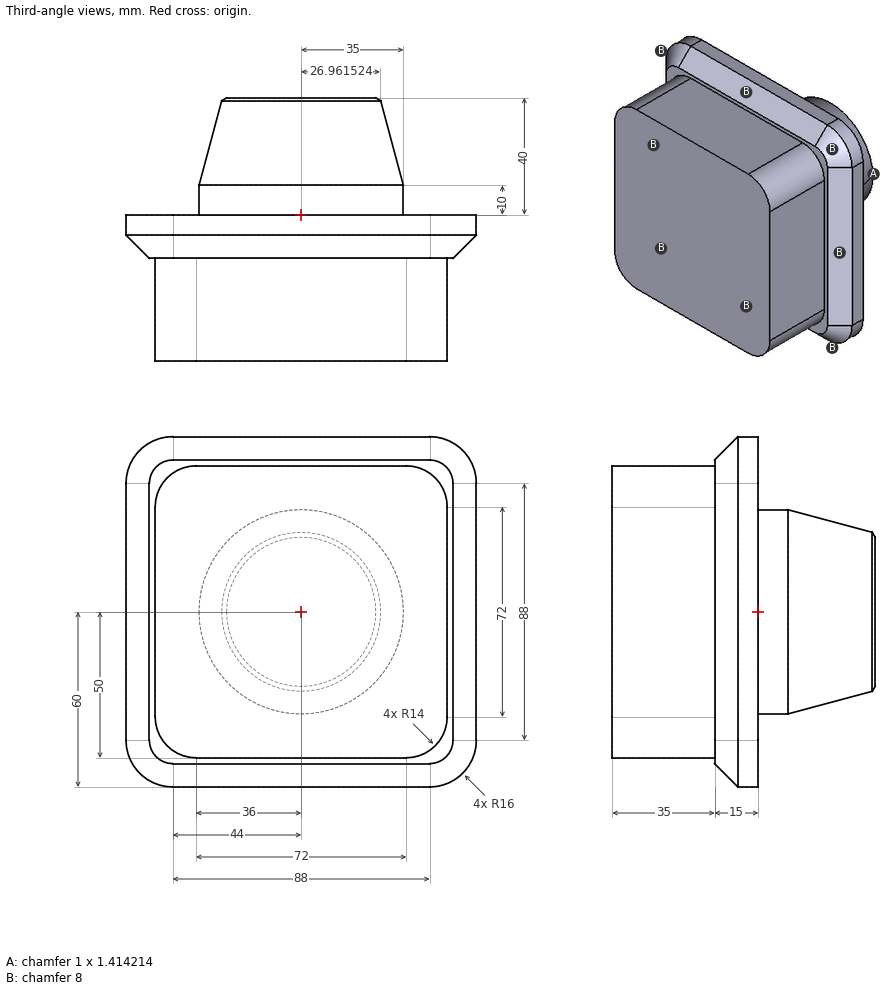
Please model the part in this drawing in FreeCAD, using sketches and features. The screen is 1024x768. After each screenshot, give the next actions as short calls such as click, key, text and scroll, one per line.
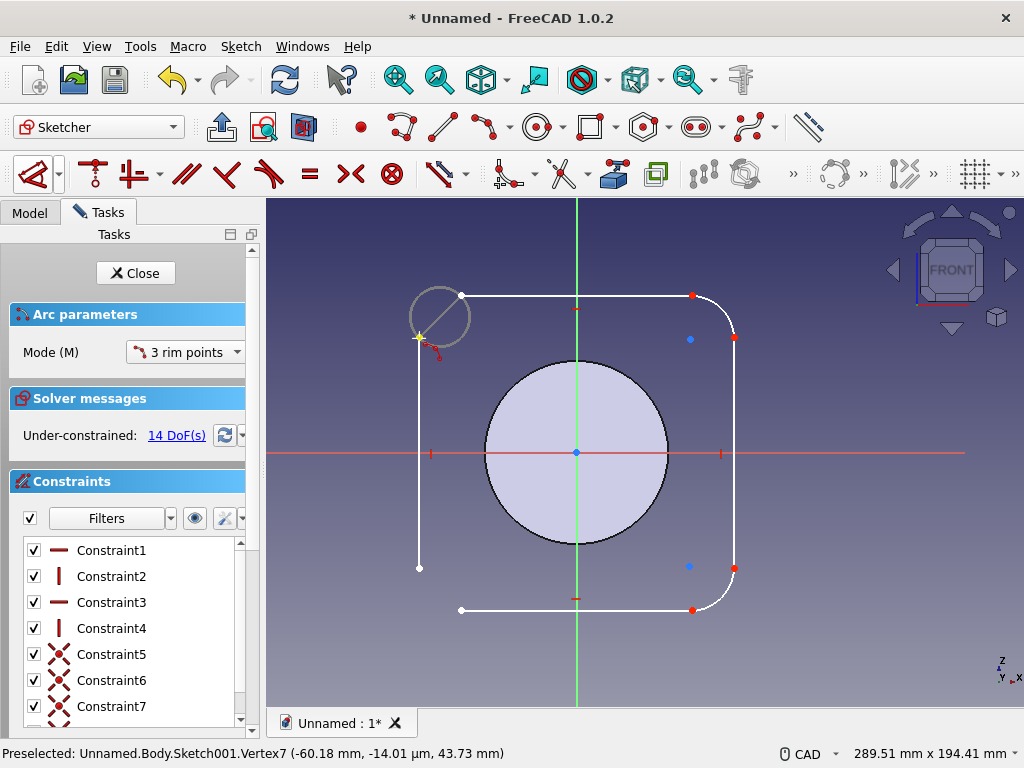
scroll(432, 308, up, 2)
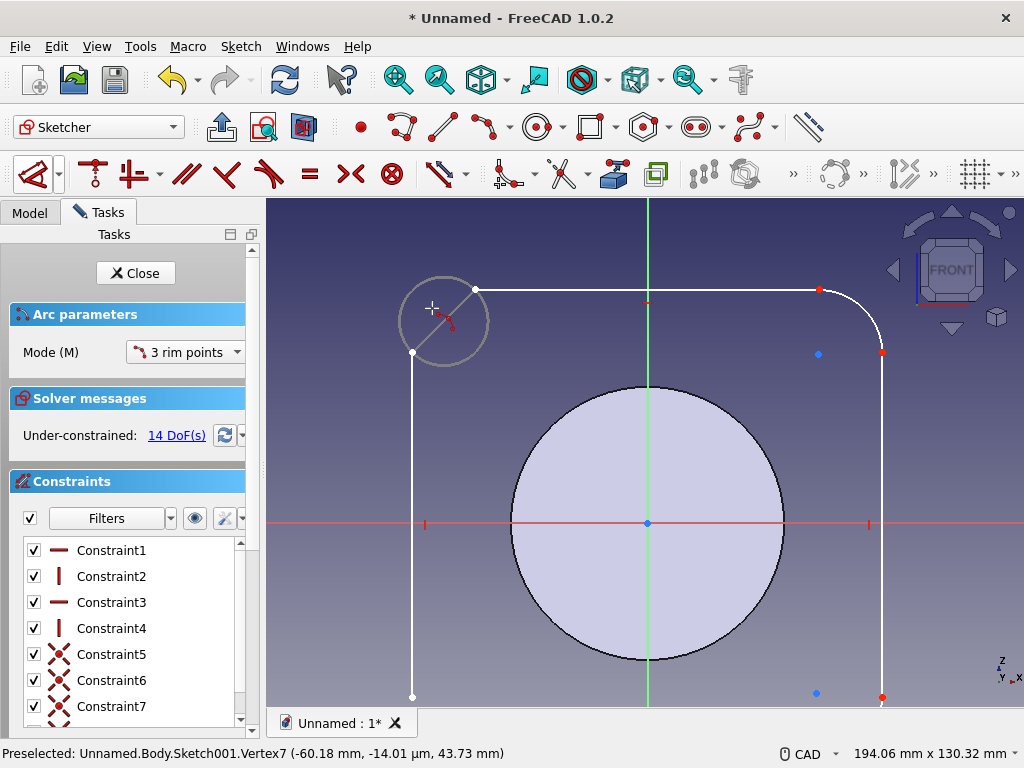
click(431, 307)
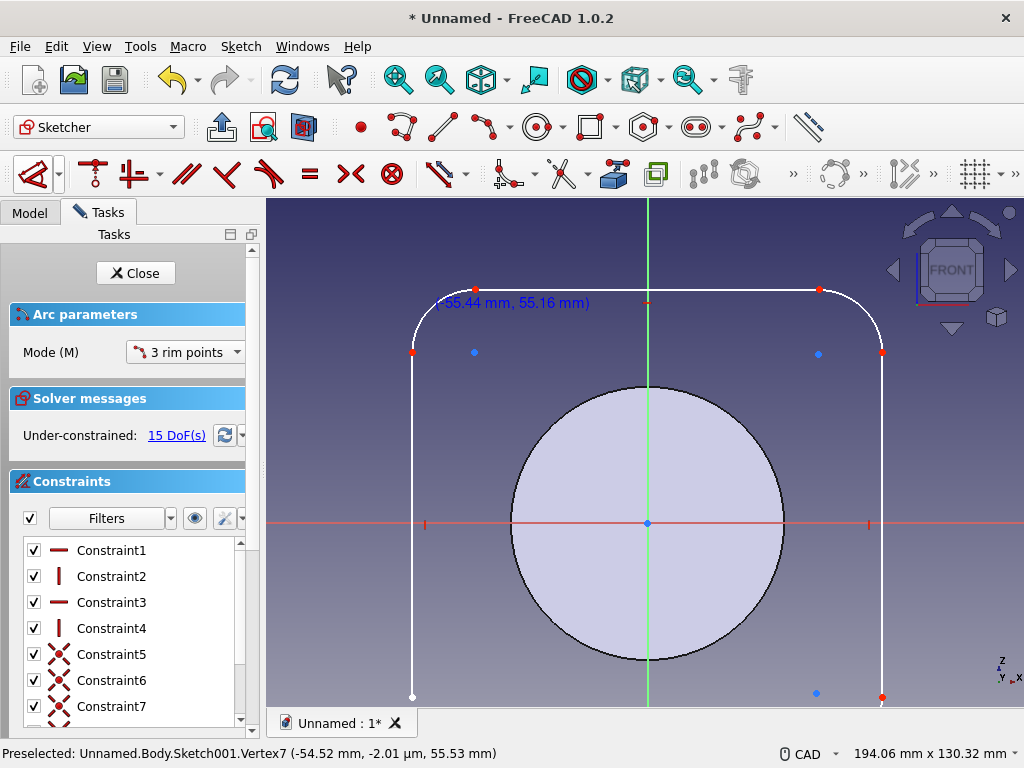
scroll(432, 308, down, 2)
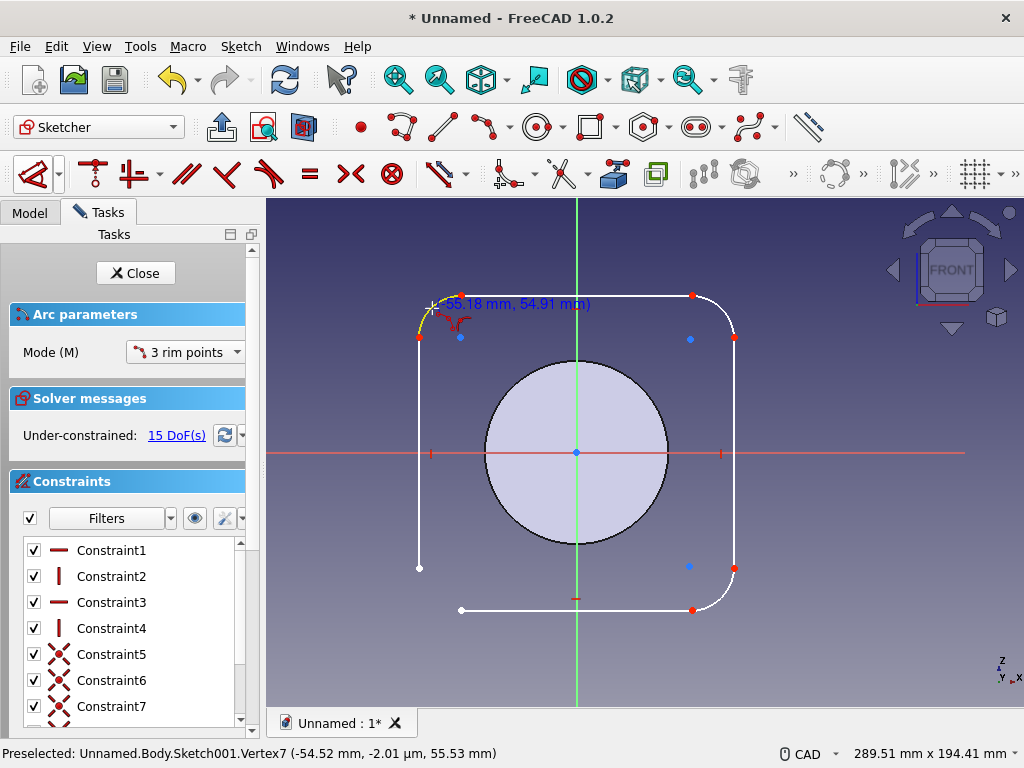
click(419, 569)
click(461, 611)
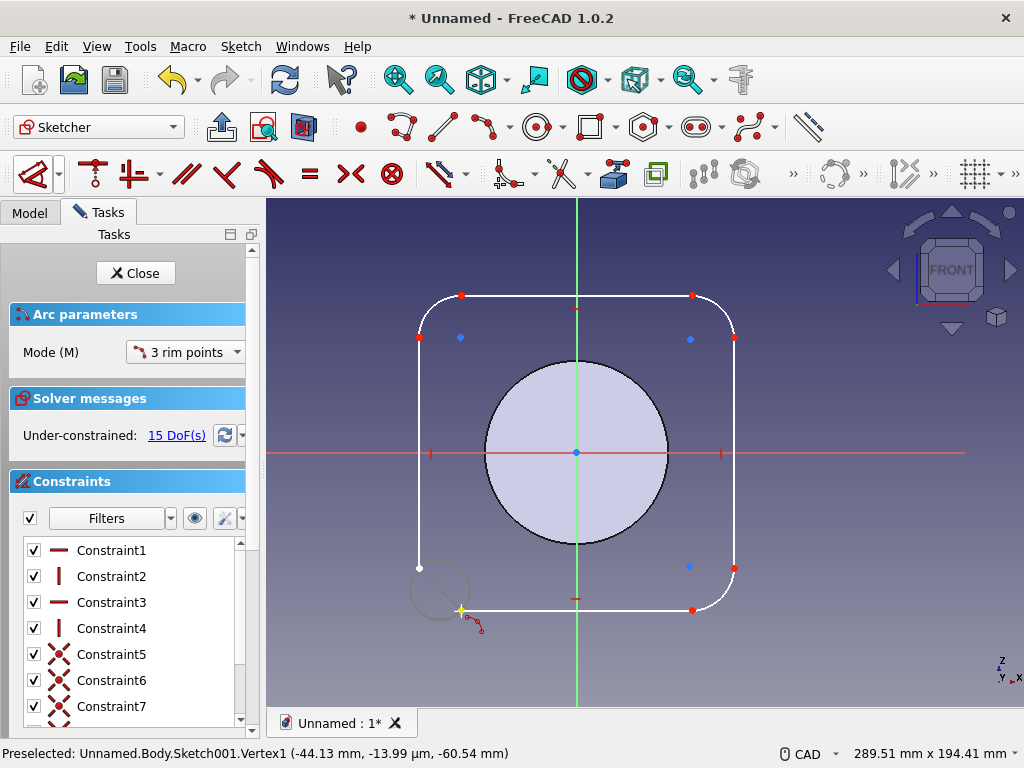
scroll(432, 597, up, 2)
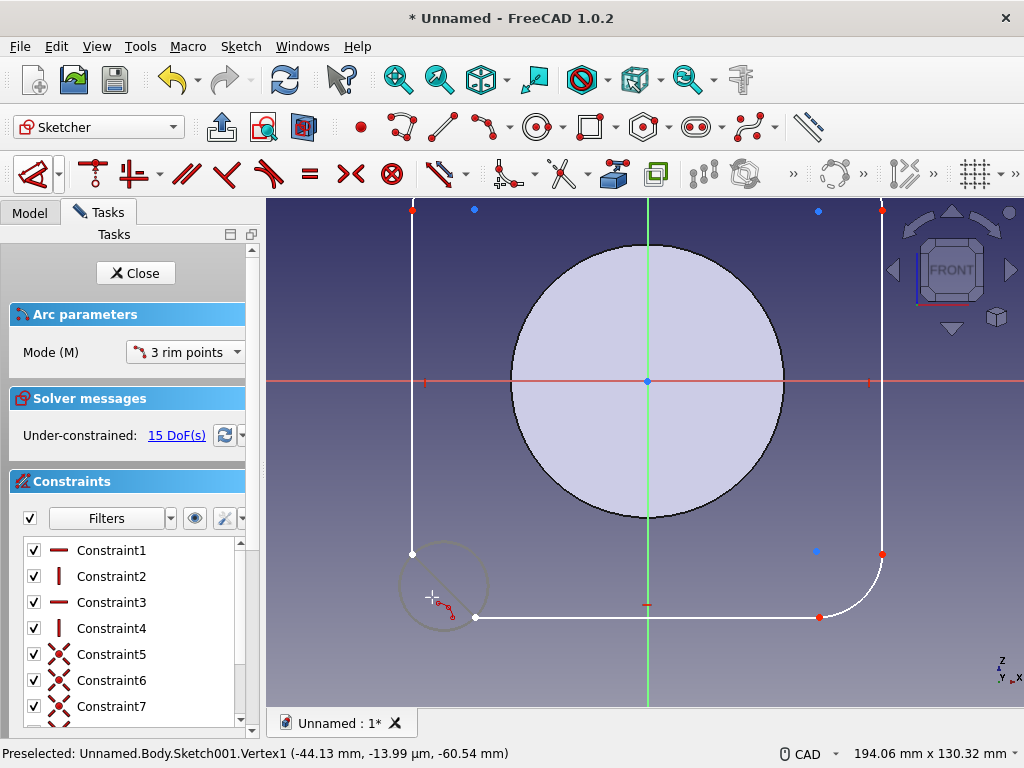
click(431, 597)
key(Escape)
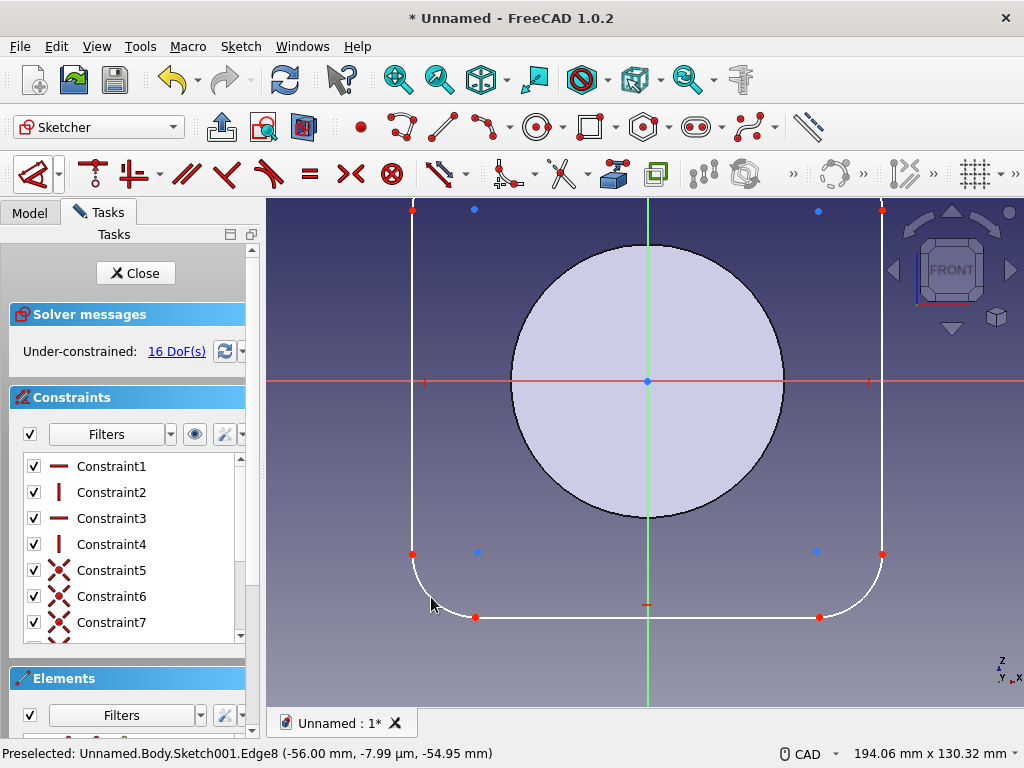
click(579, 617)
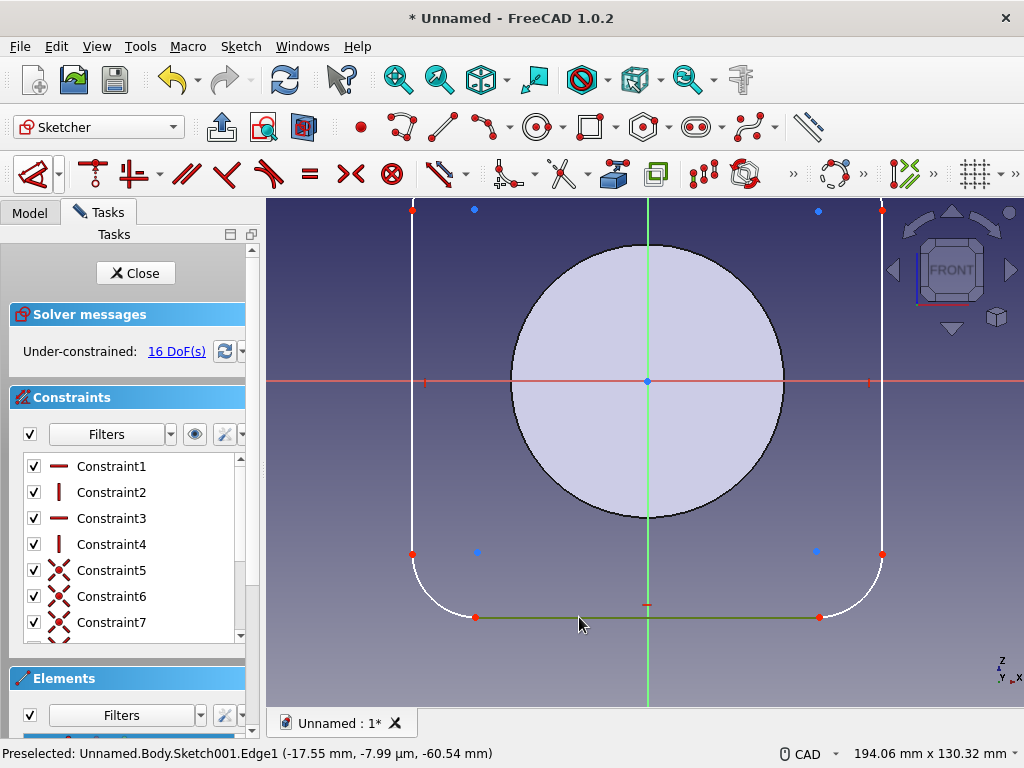
click(848, 610)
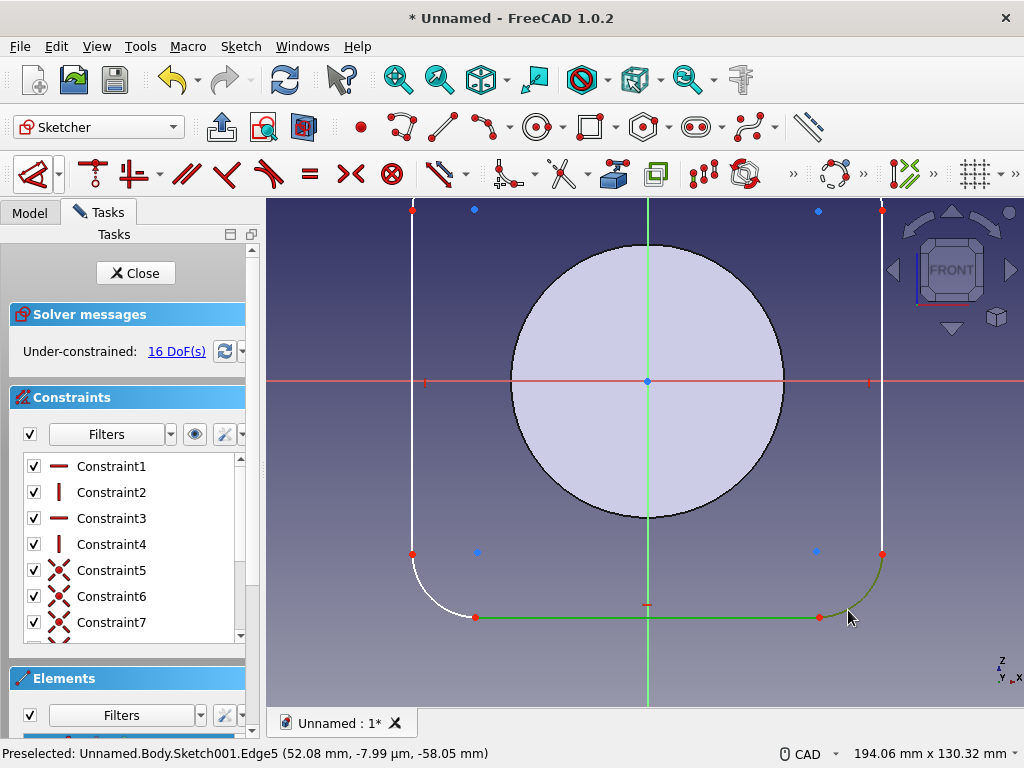
key(t)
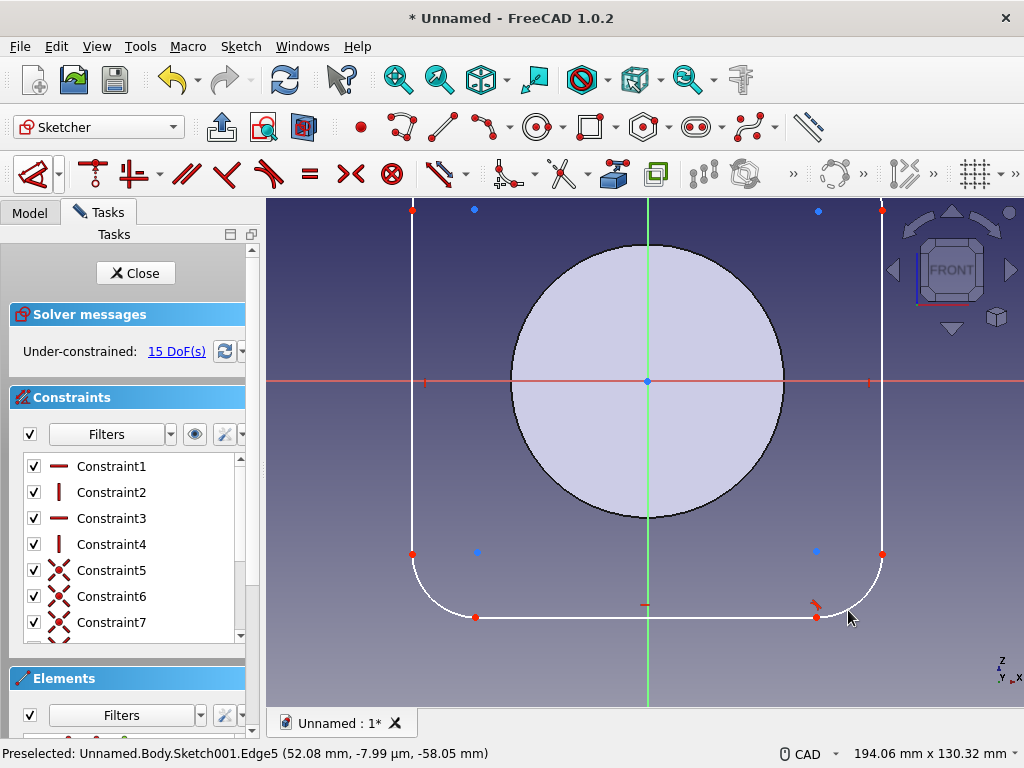
click(578, 618)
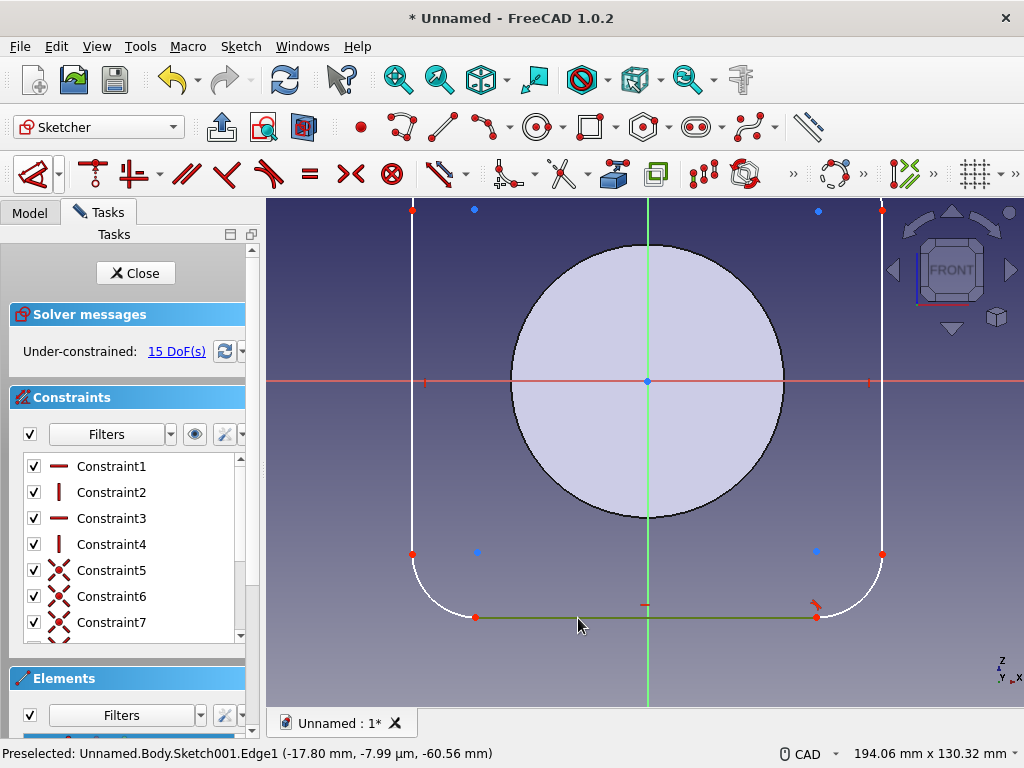
click(420, 583)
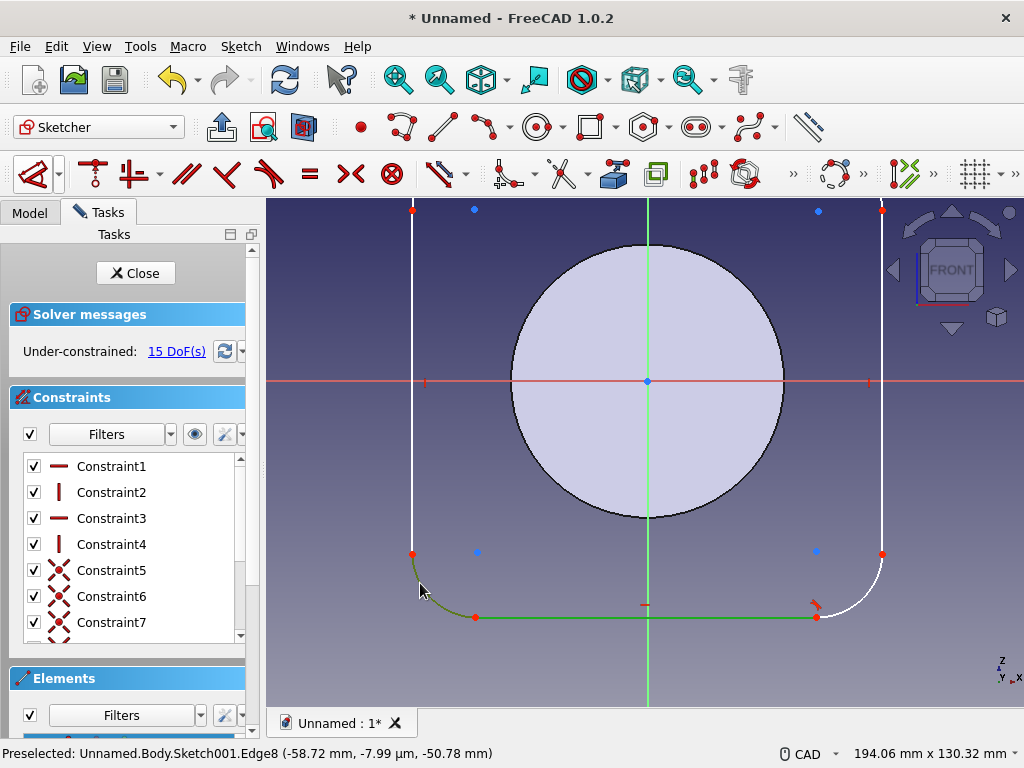
key(t)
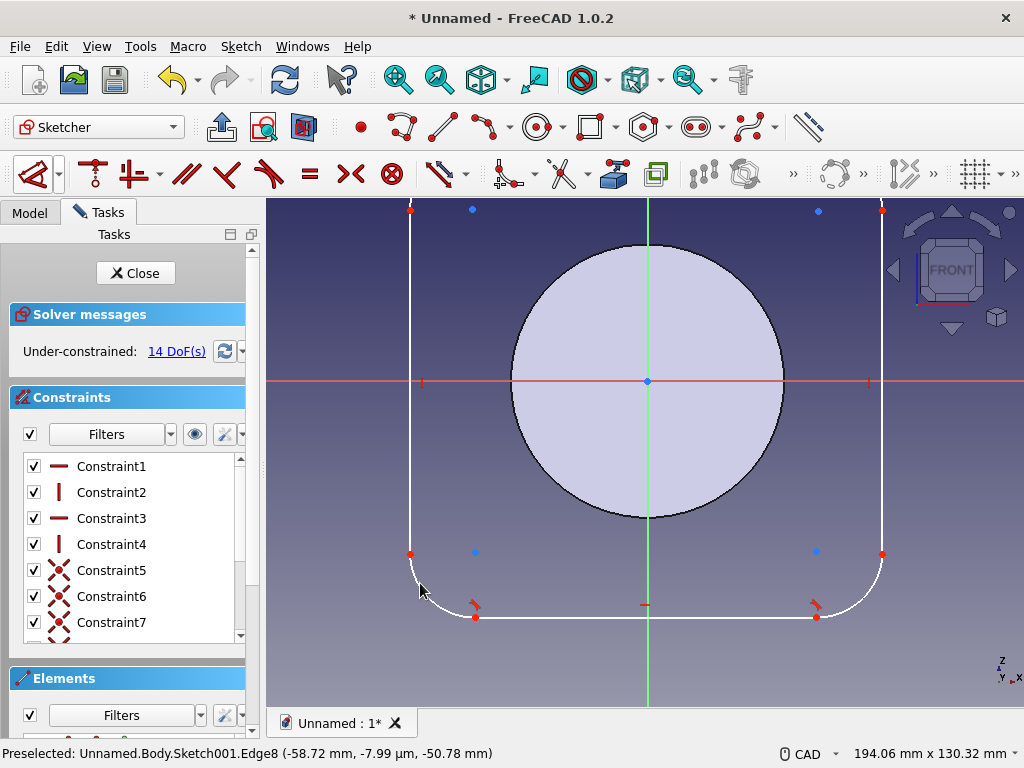
scroll(432, 598, down, 2)